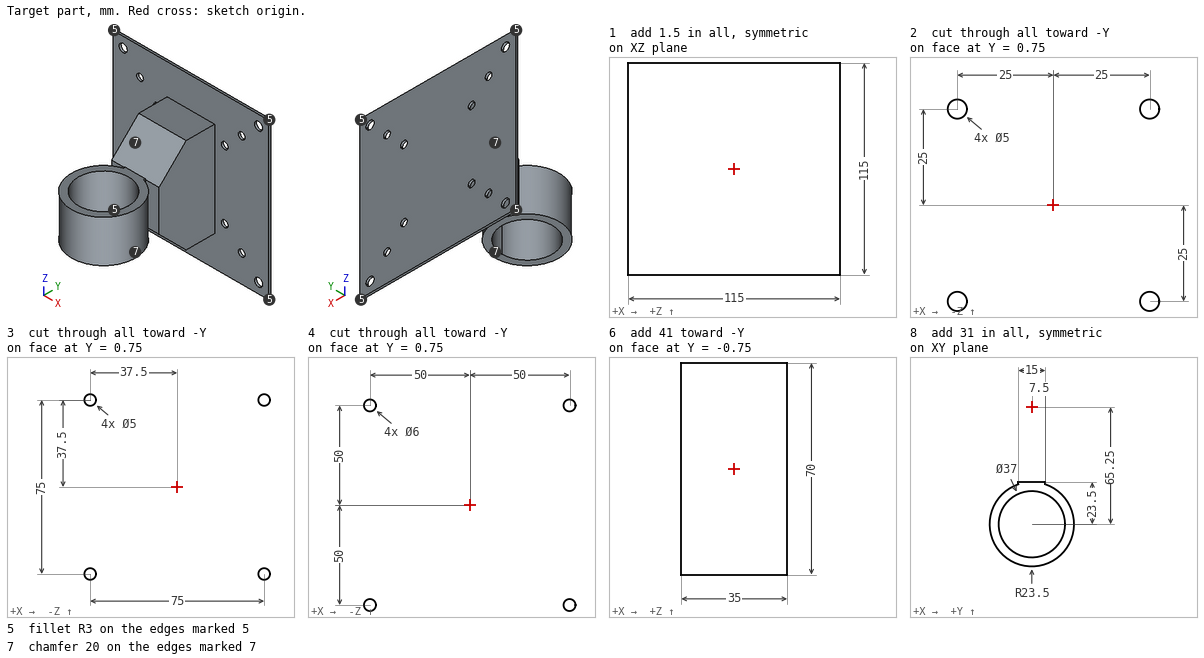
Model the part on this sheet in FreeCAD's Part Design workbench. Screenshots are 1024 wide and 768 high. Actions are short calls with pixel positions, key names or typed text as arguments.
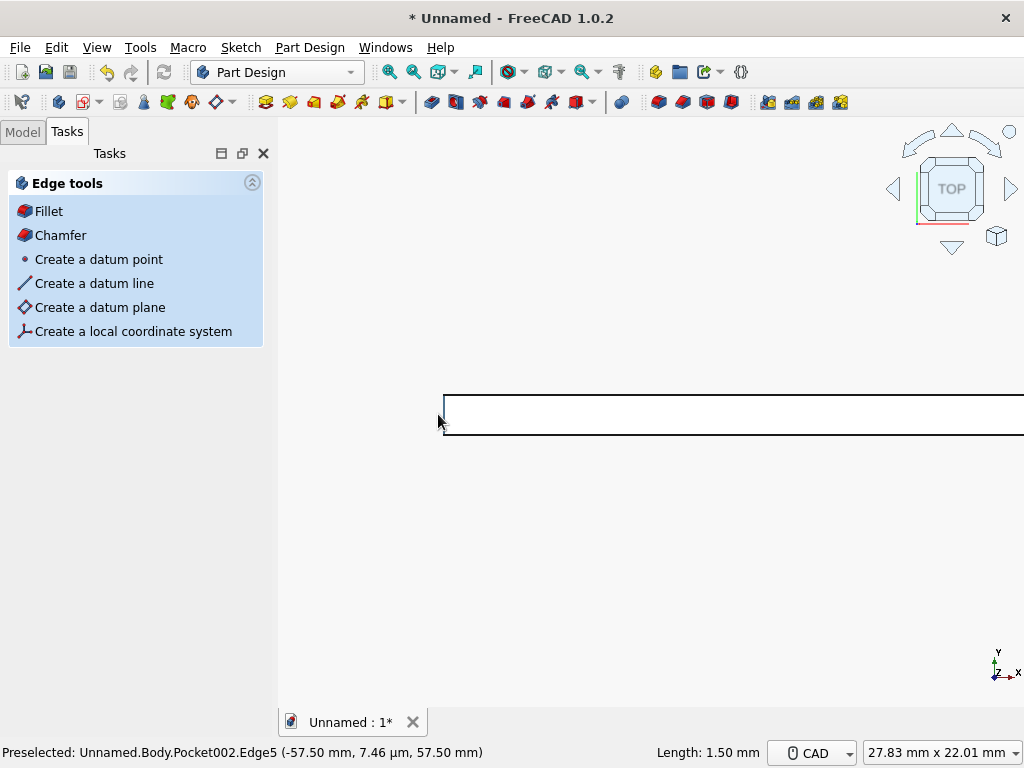
click(390, 72)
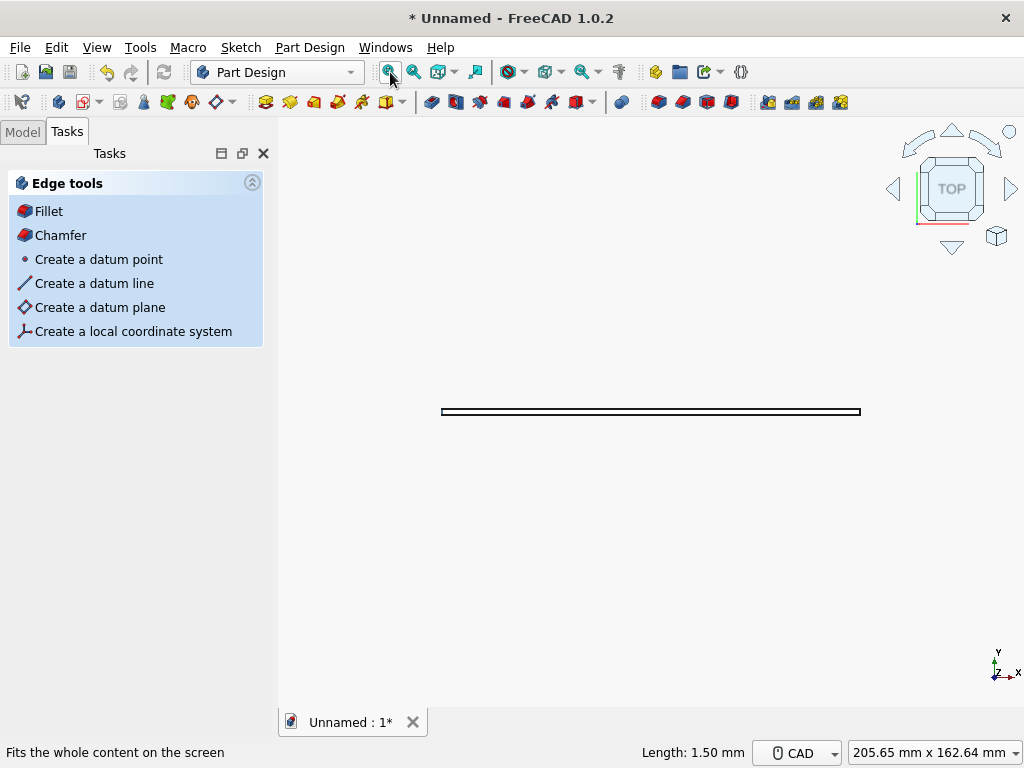
key(1)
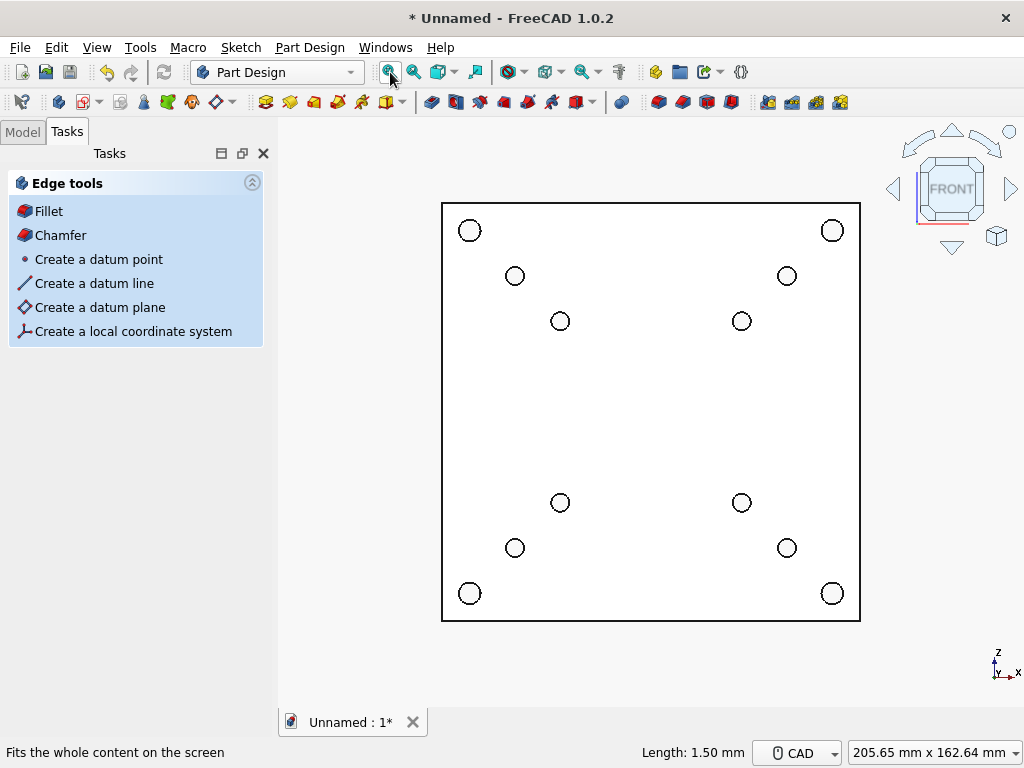
scroll(442, 620, up, 10)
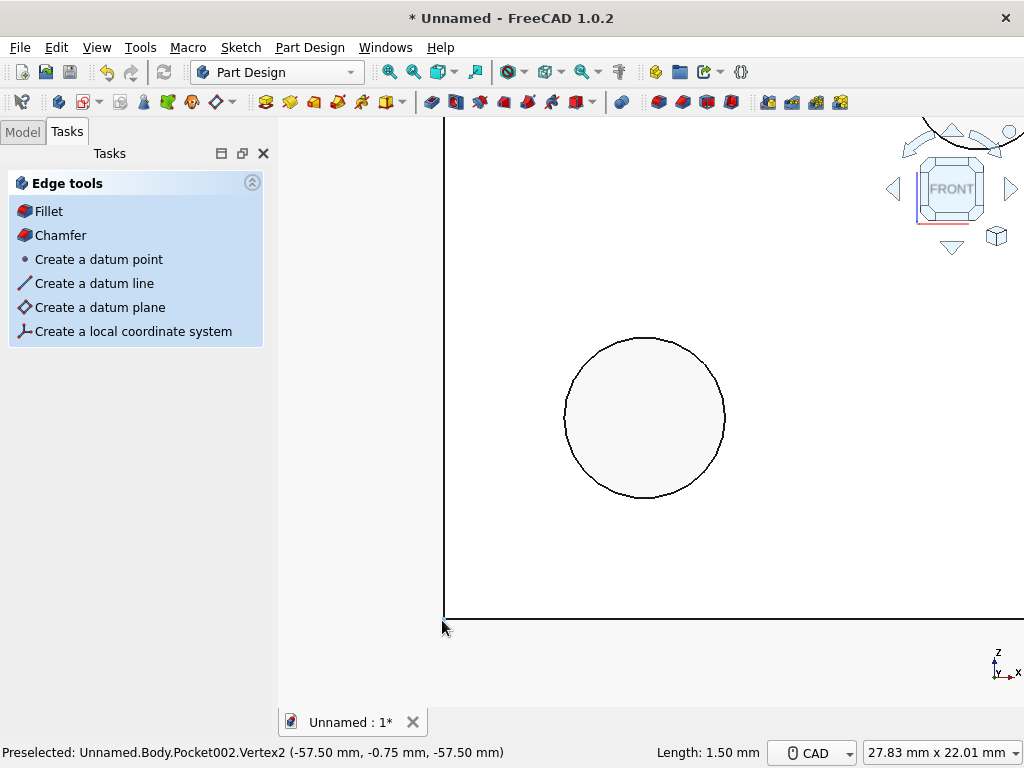
key(v)
key(f)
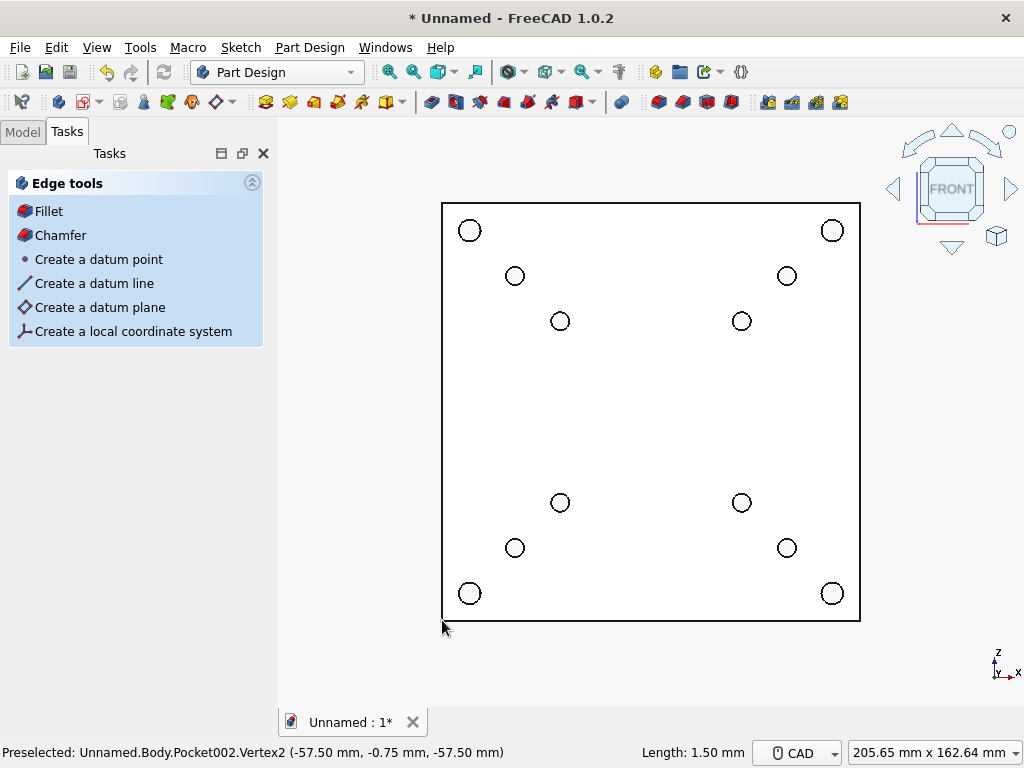
key(3)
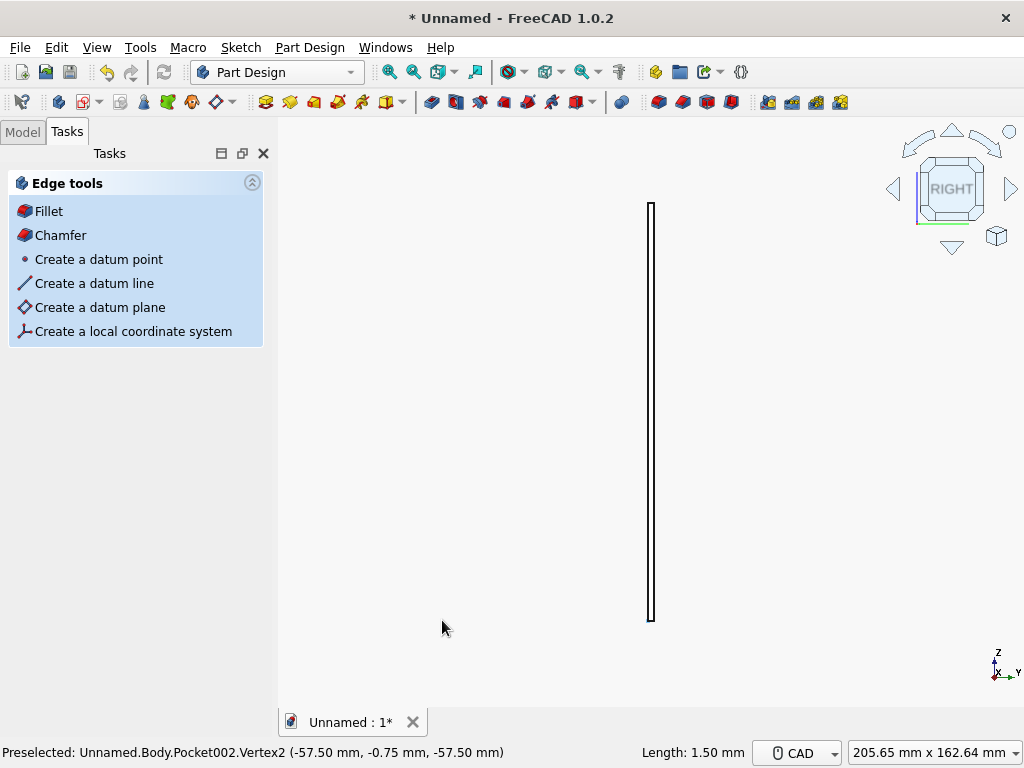
scroll(651, 620, up, 10)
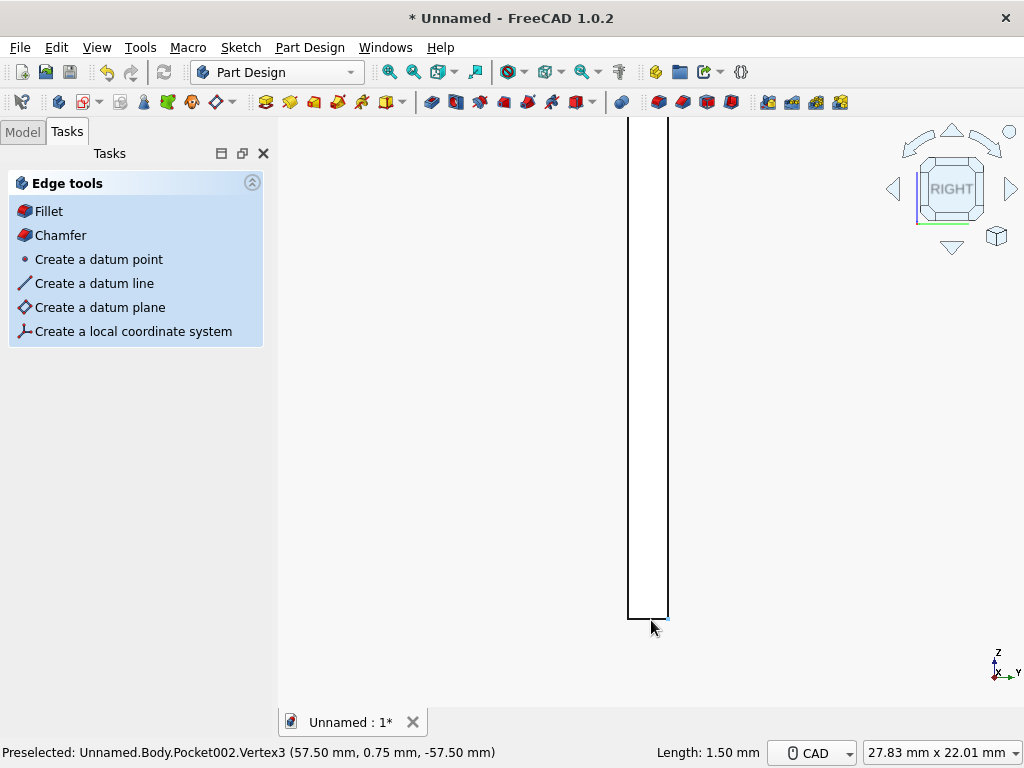
click(648, 618, ctrl)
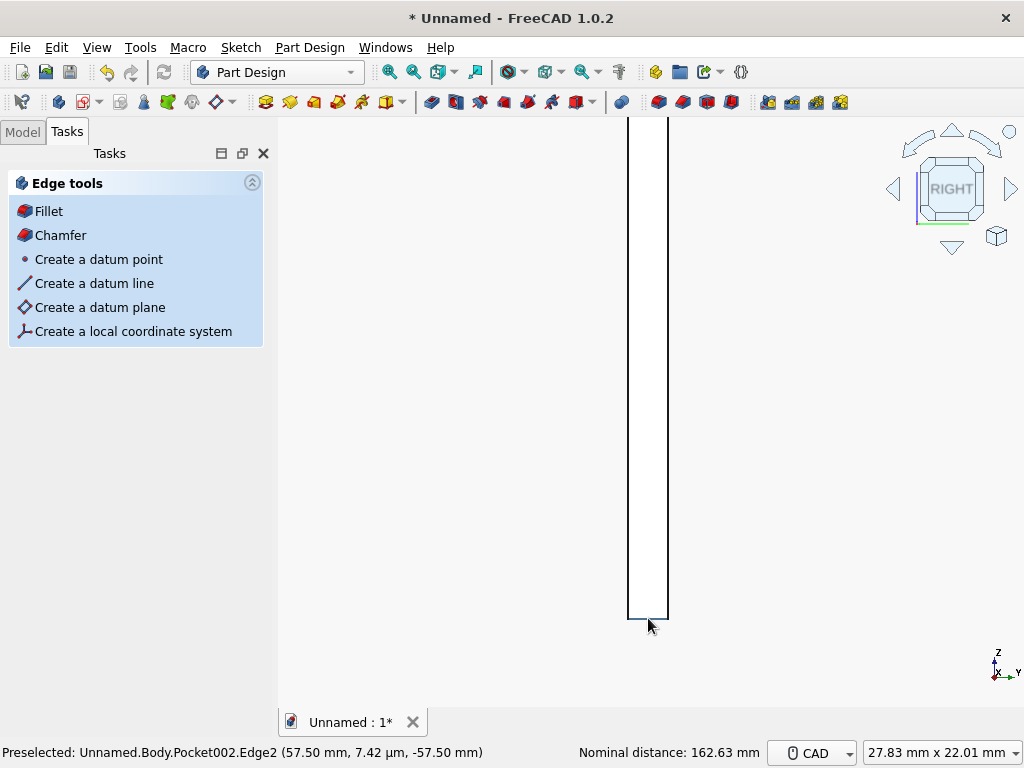
click(390, 72)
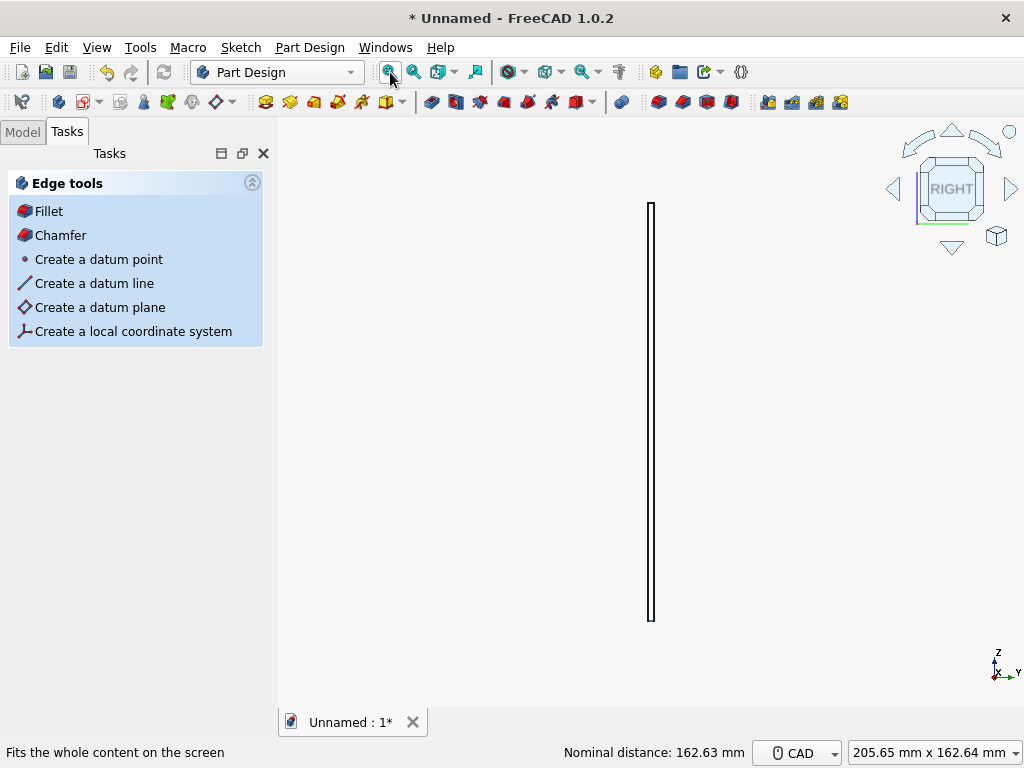
key(5)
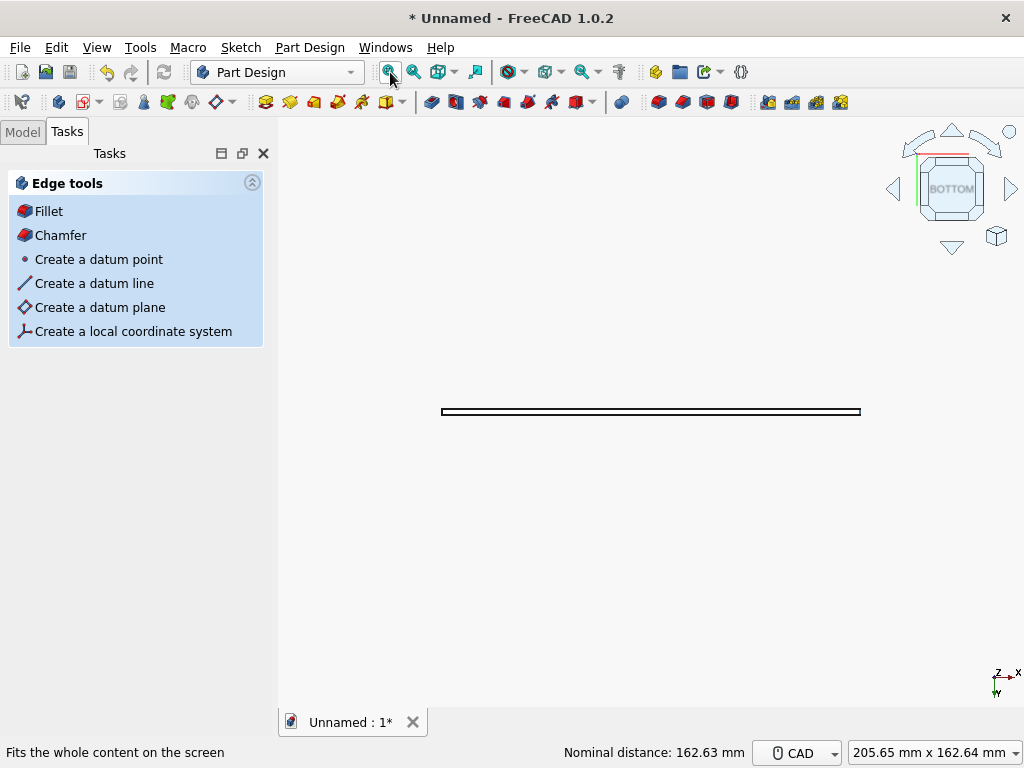
scroll(442, 411, up, 10)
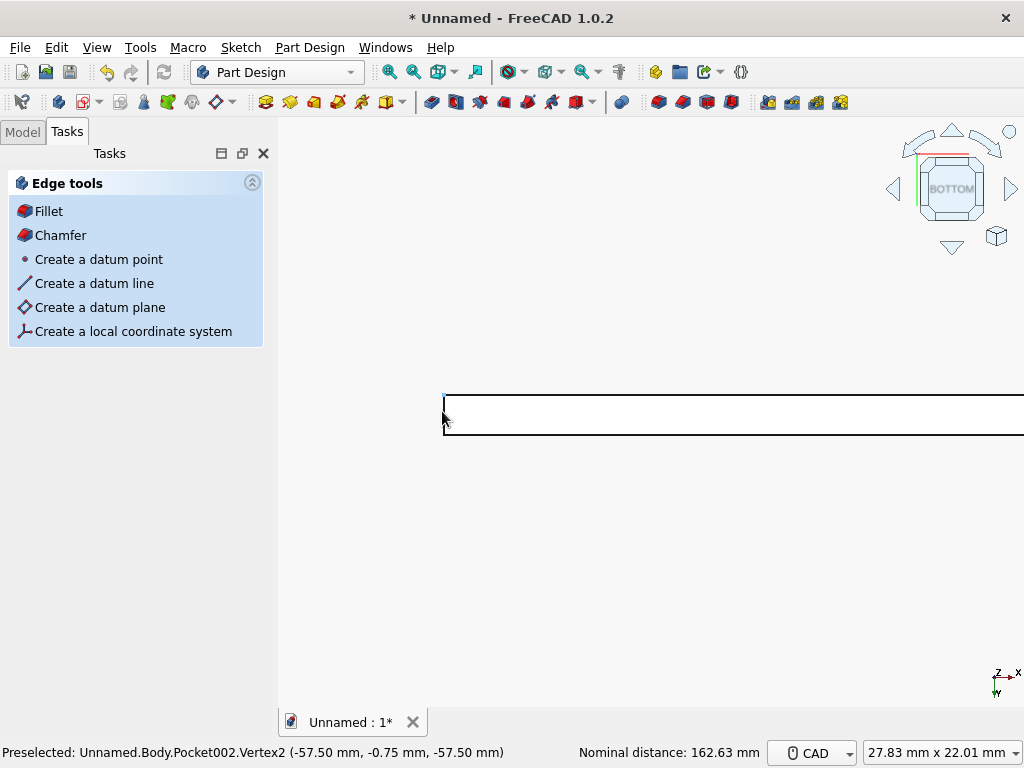
click(444, 414, ctrl)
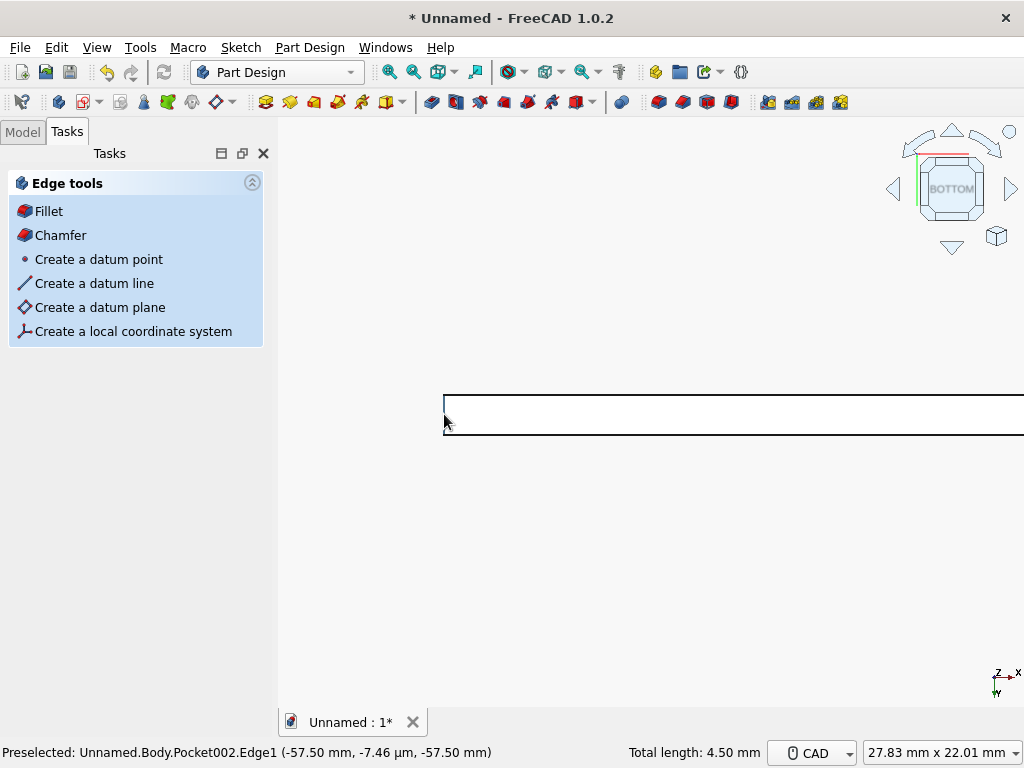
key(v)
key(f)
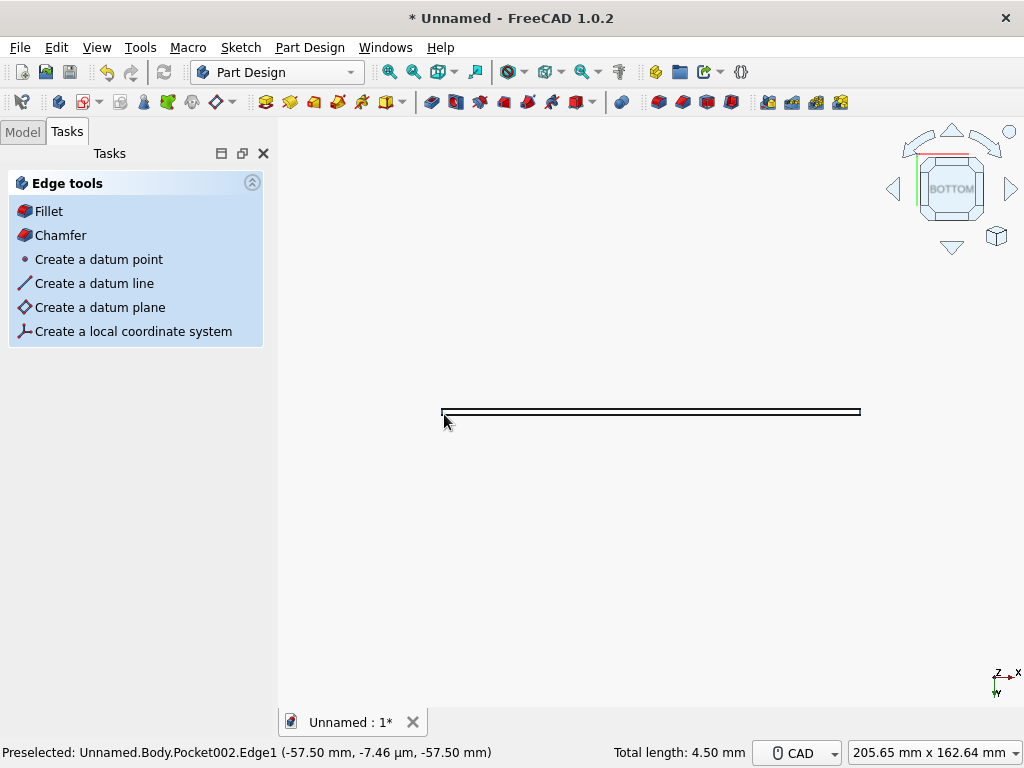
key(4)